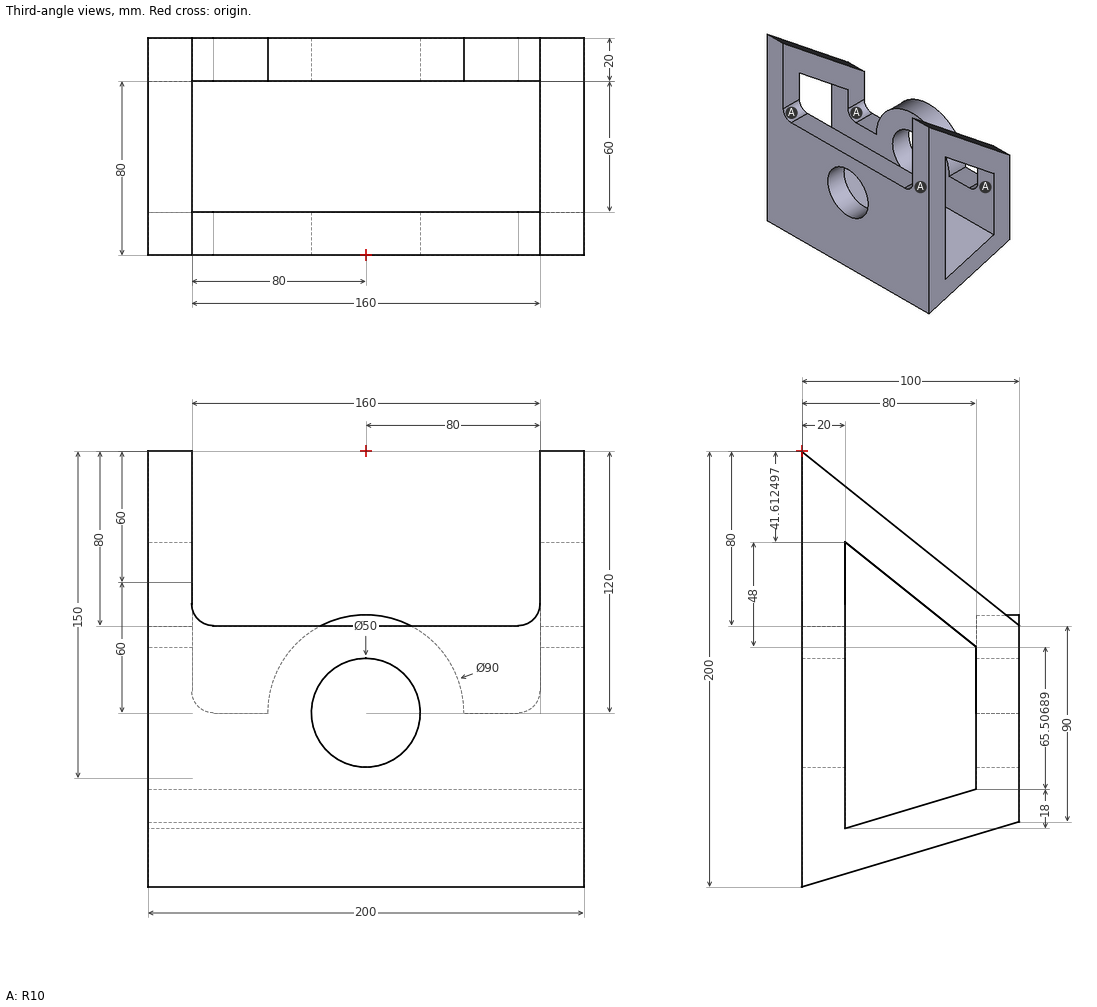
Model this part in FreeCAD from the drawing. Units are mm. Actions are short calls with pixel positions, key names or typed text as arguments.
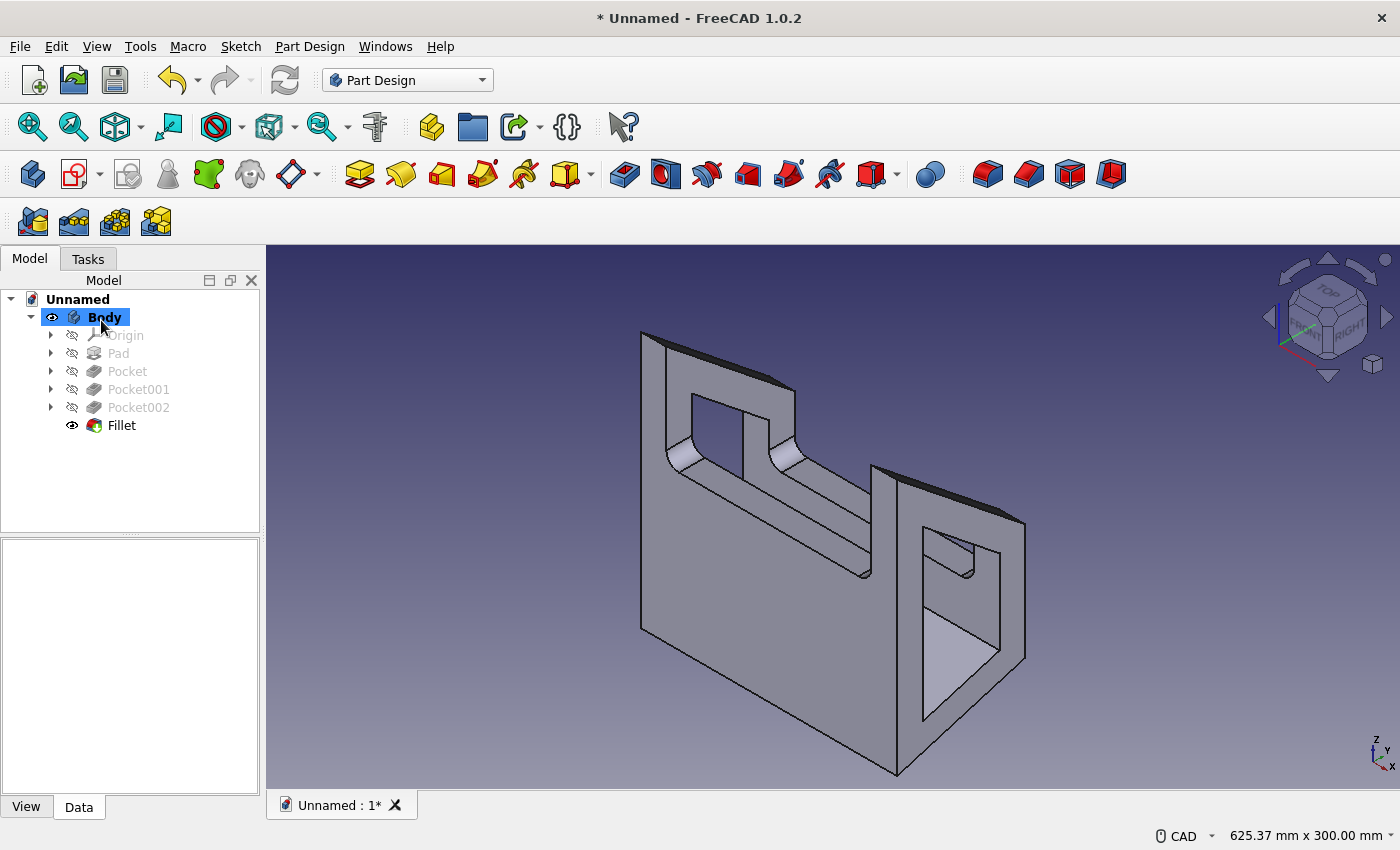
key(4)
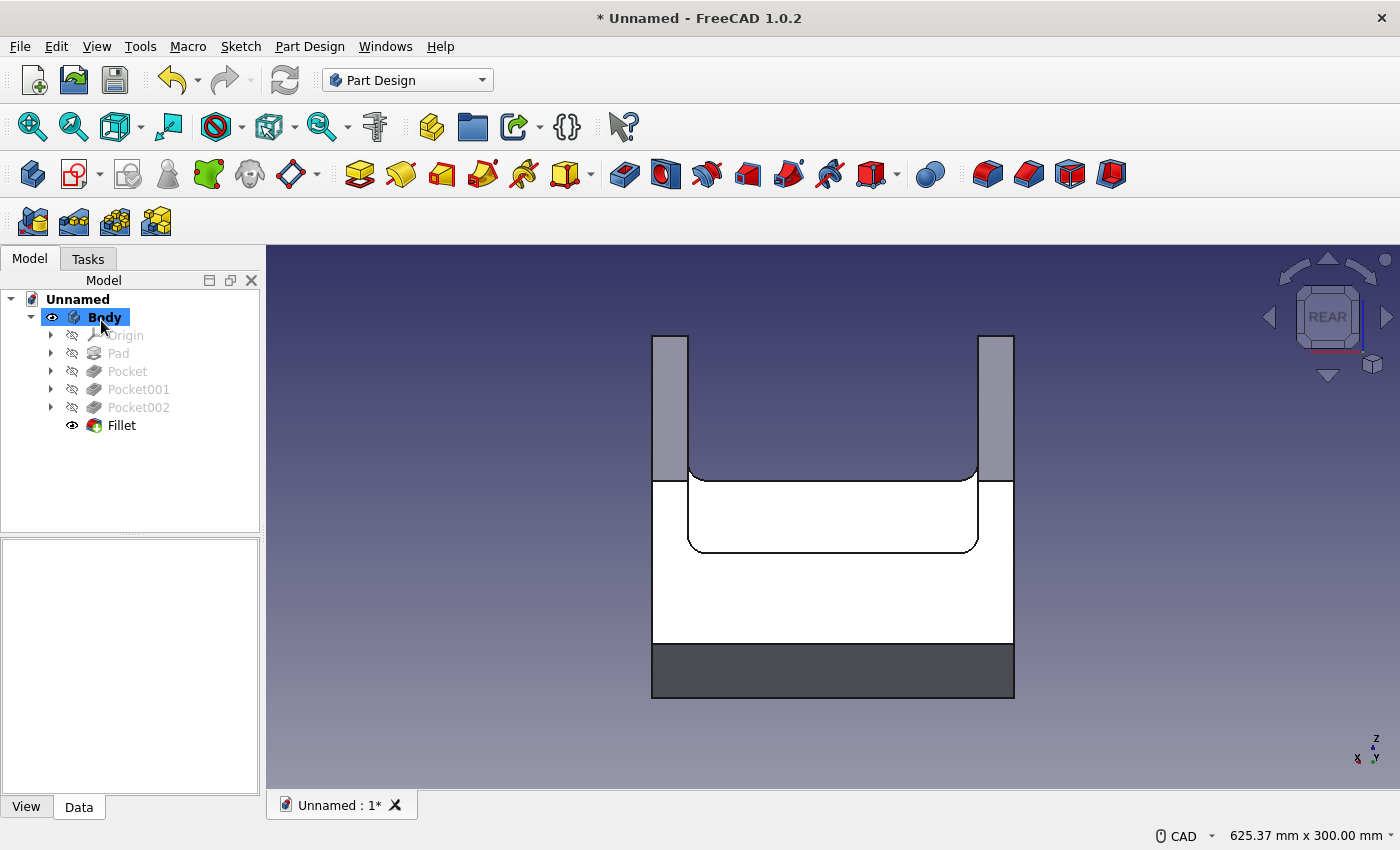
click(729, 608)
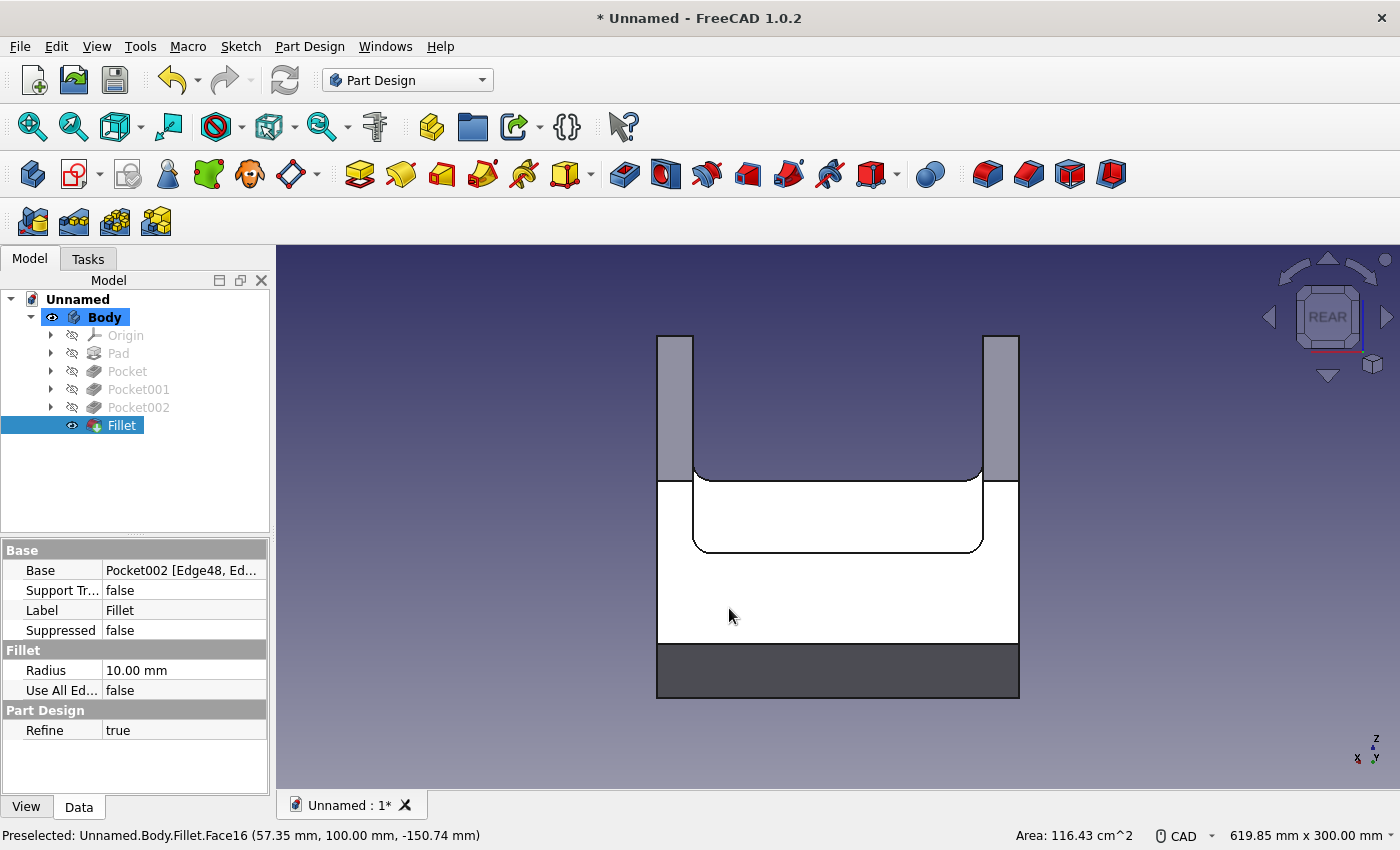
click(74, 174)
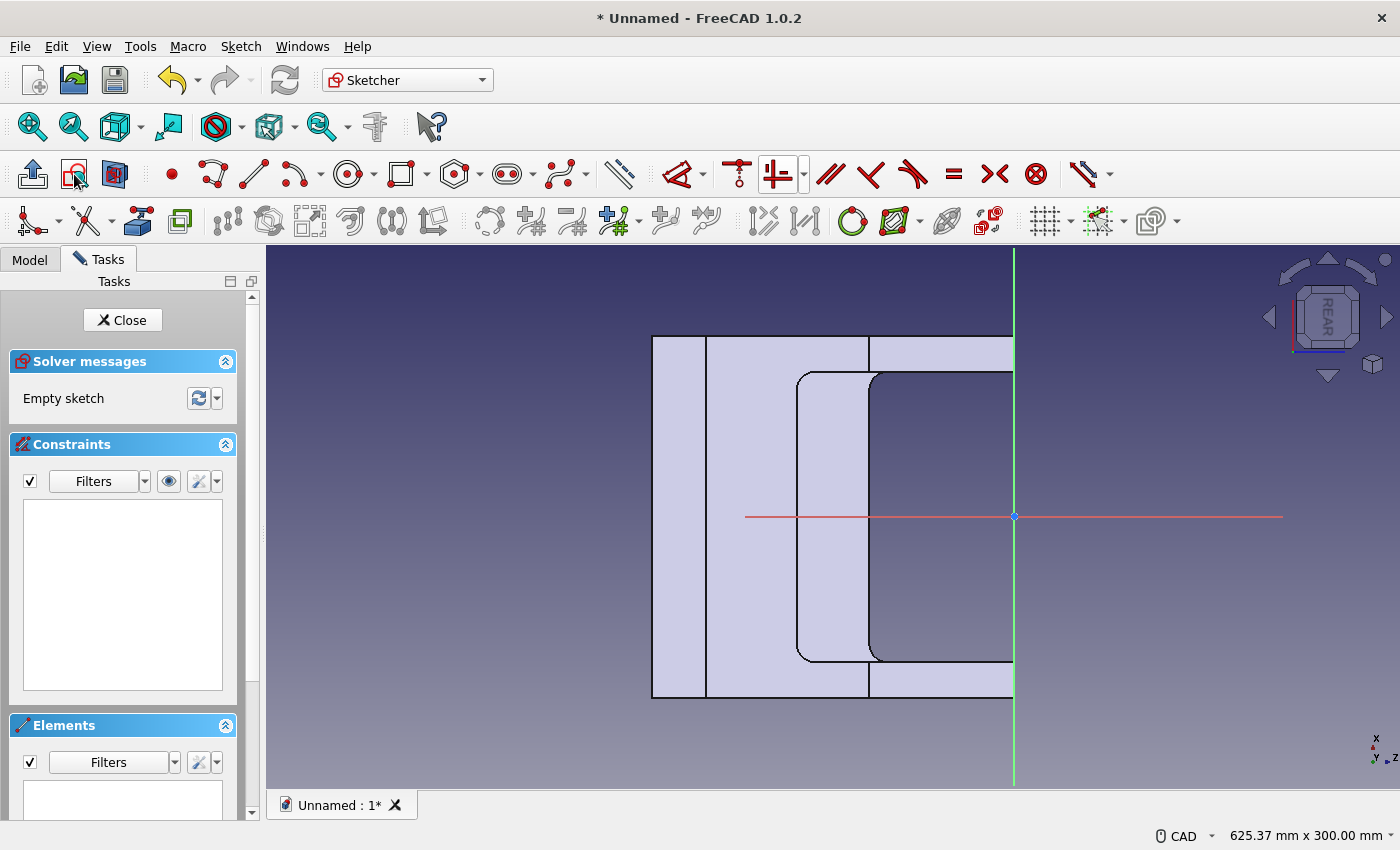
scroll(947, 517, up, 4)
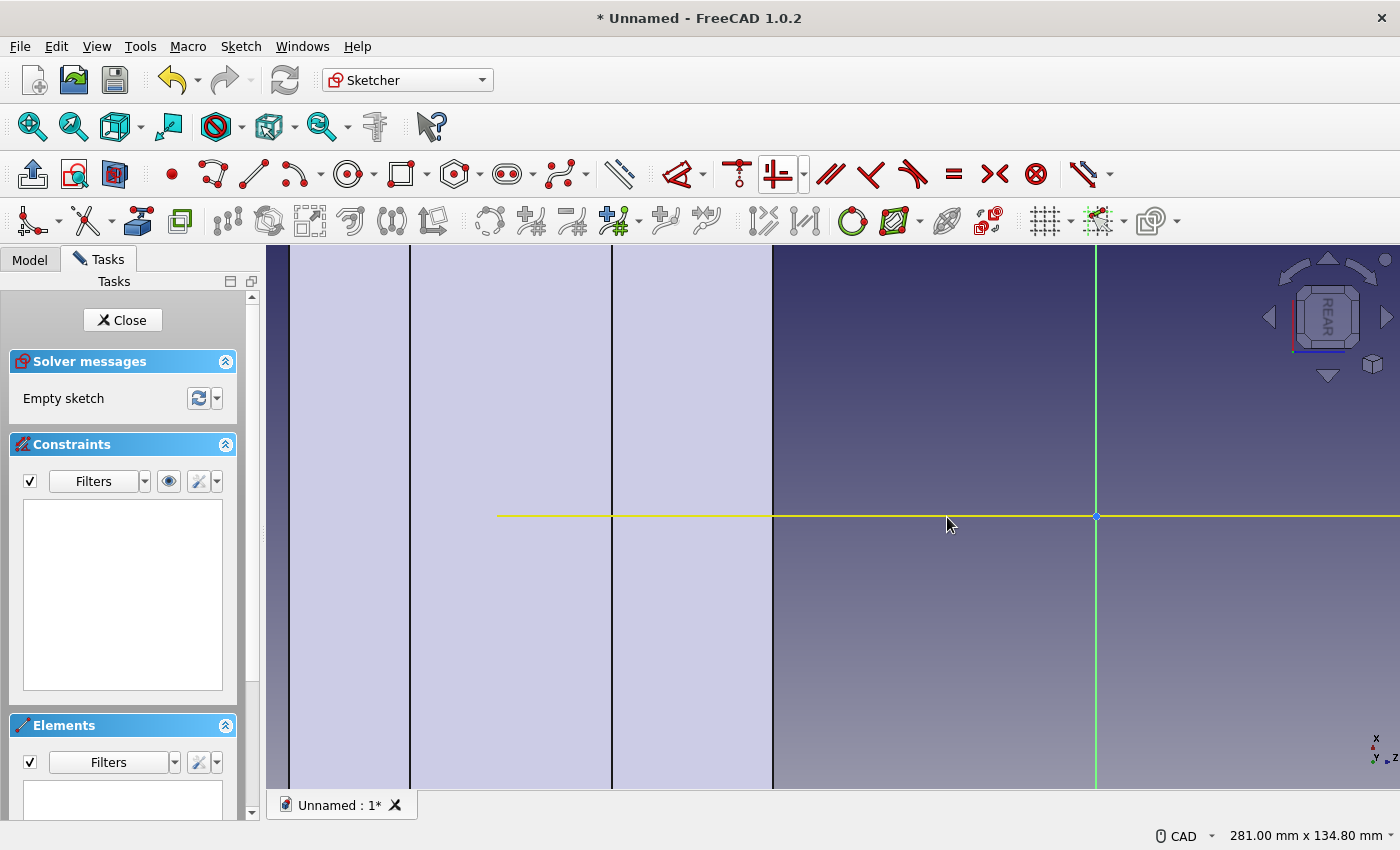
key(g)
key(c)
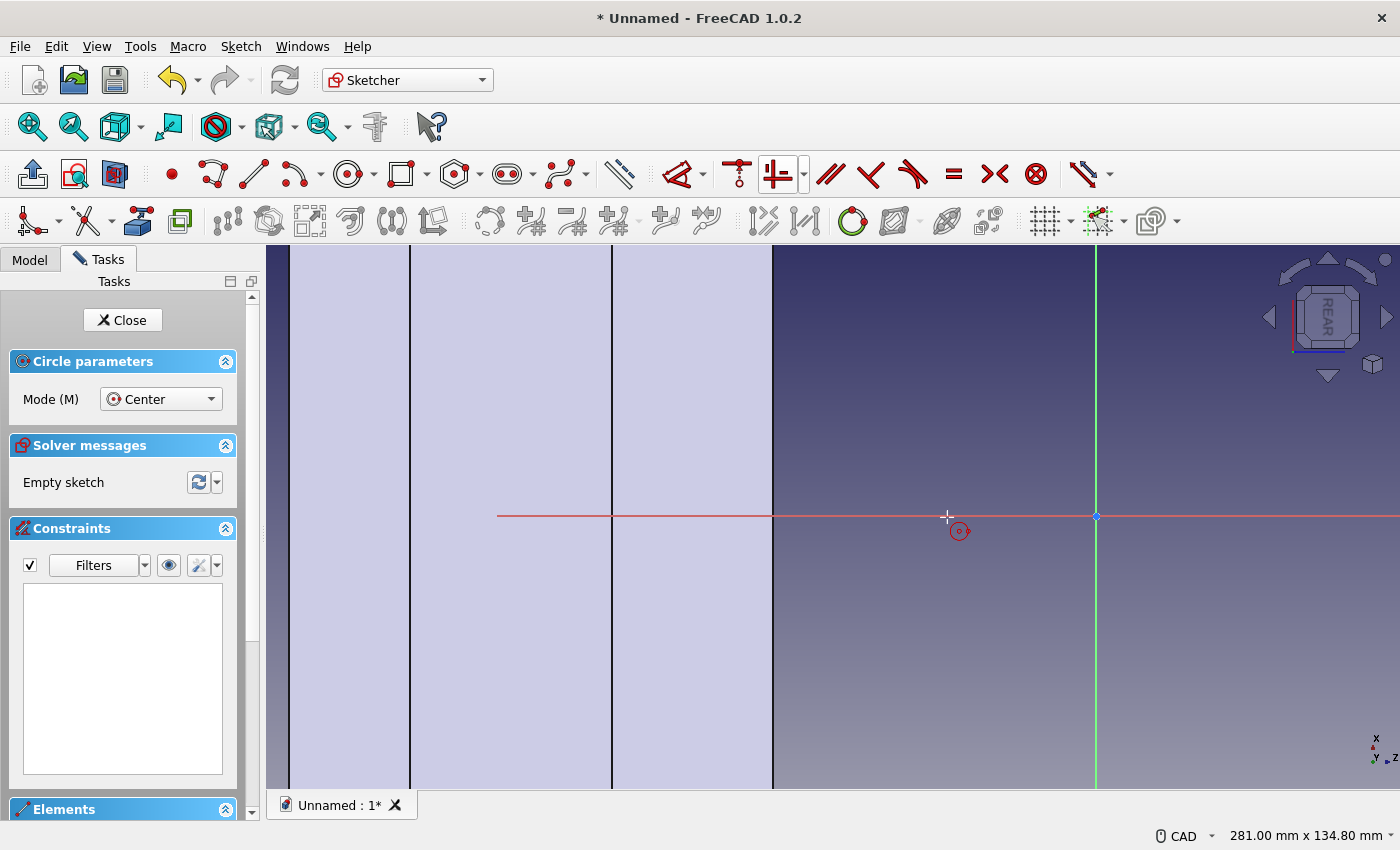
click(612, 516)
move(740, 388)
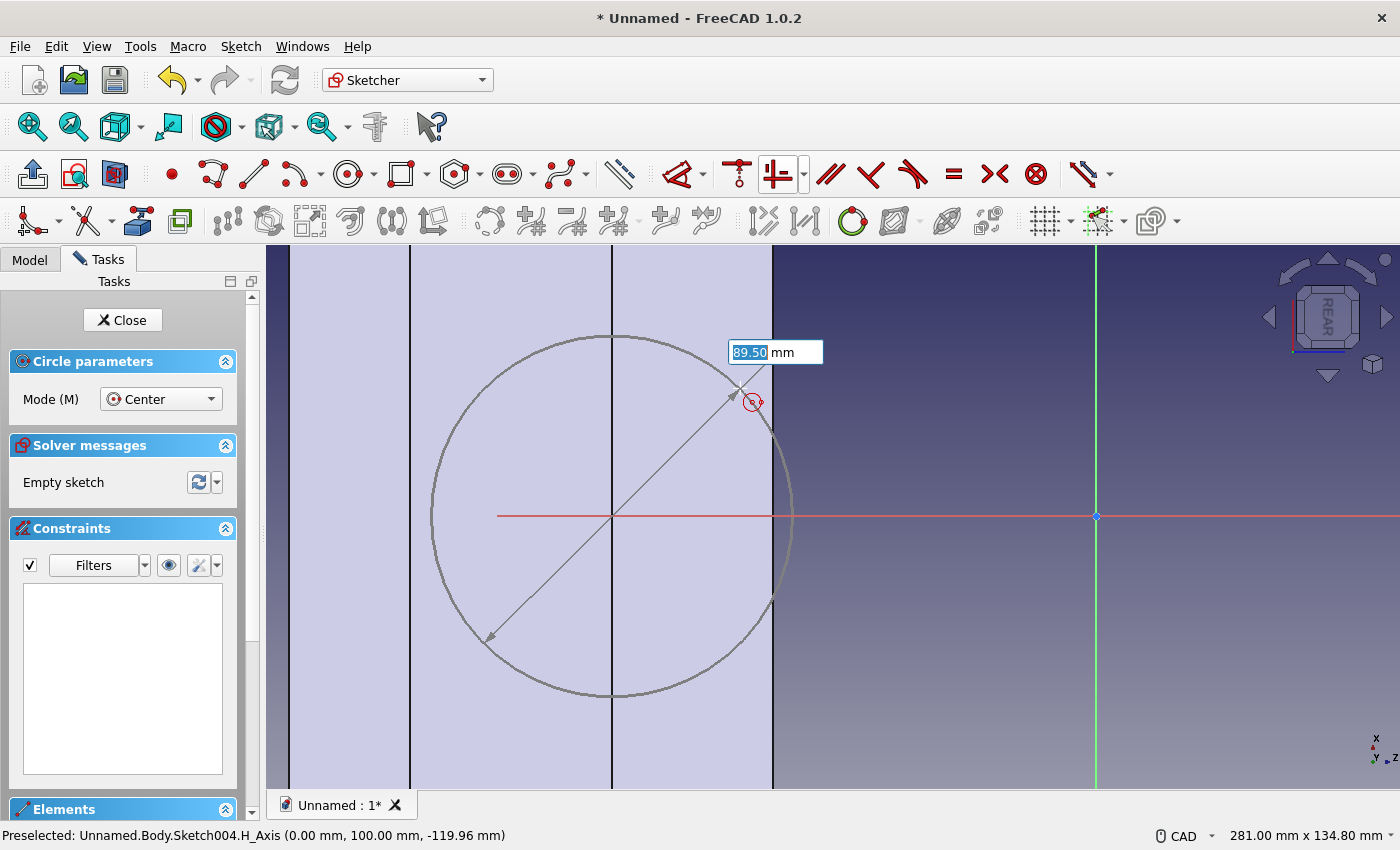
text(90)
key(Return)
key(Escape)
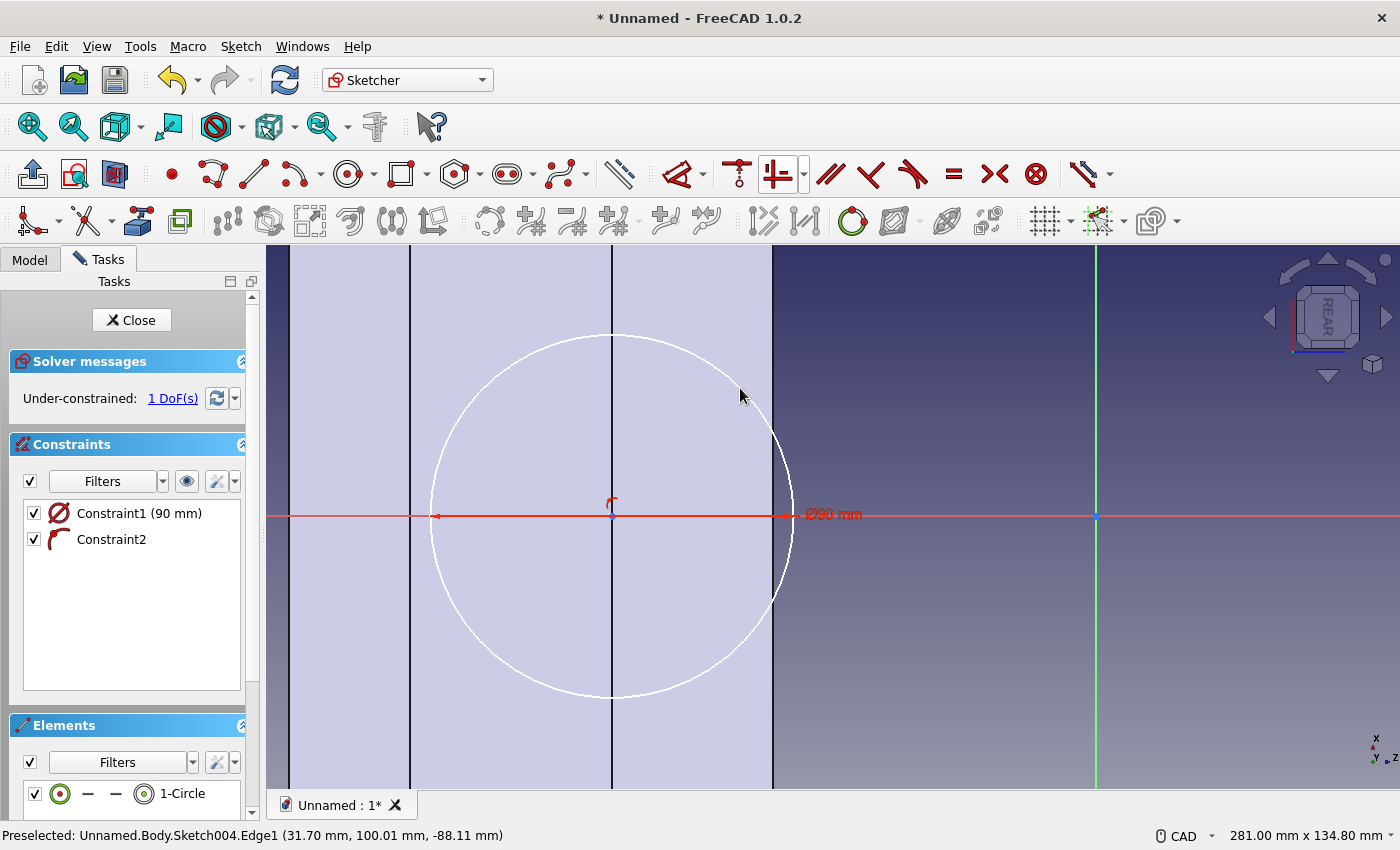
key(d)